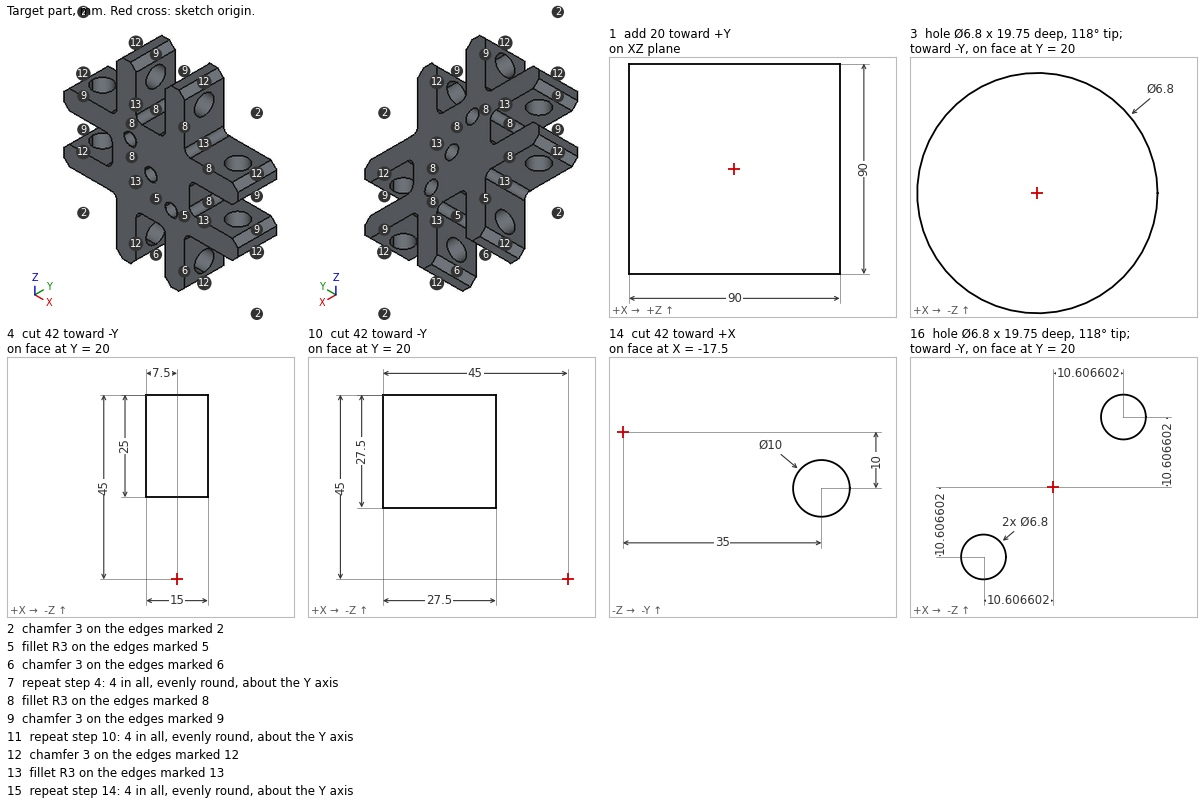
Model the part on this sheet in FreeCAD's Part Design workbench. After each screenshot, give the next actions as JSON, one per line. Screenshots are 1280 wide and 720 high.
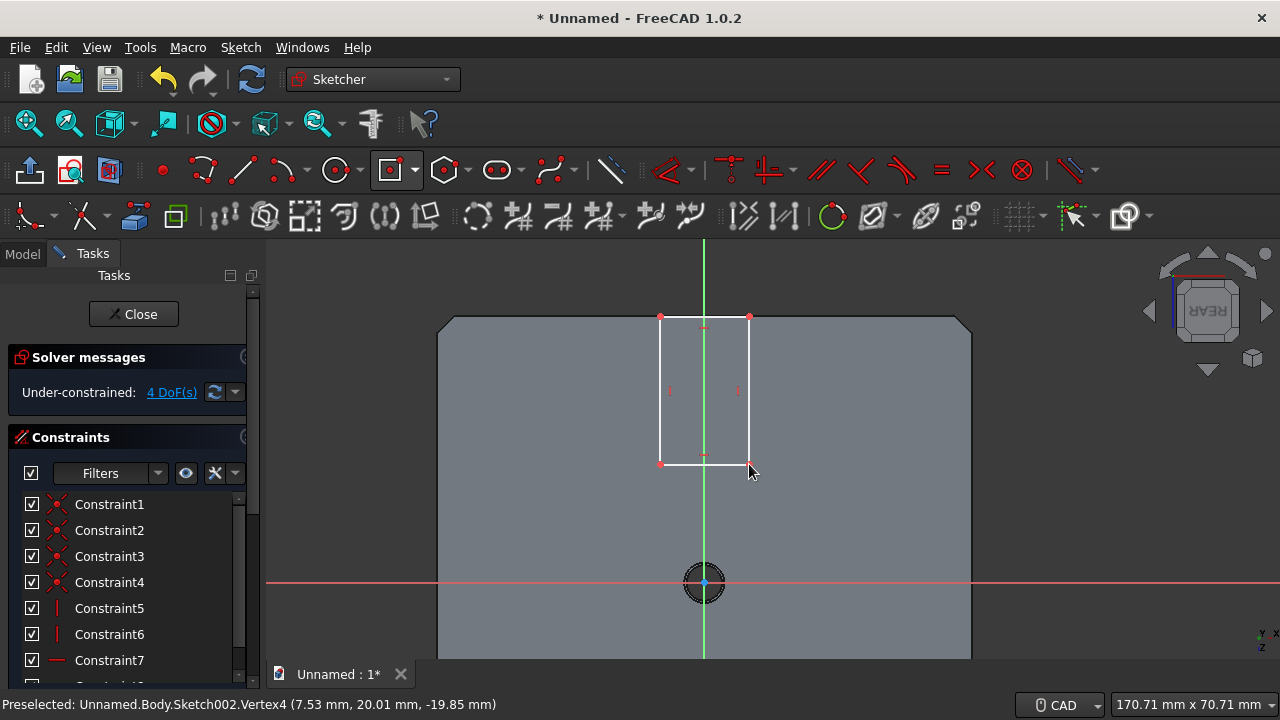
{"action": "left_click", "coordinate": [666, 170]}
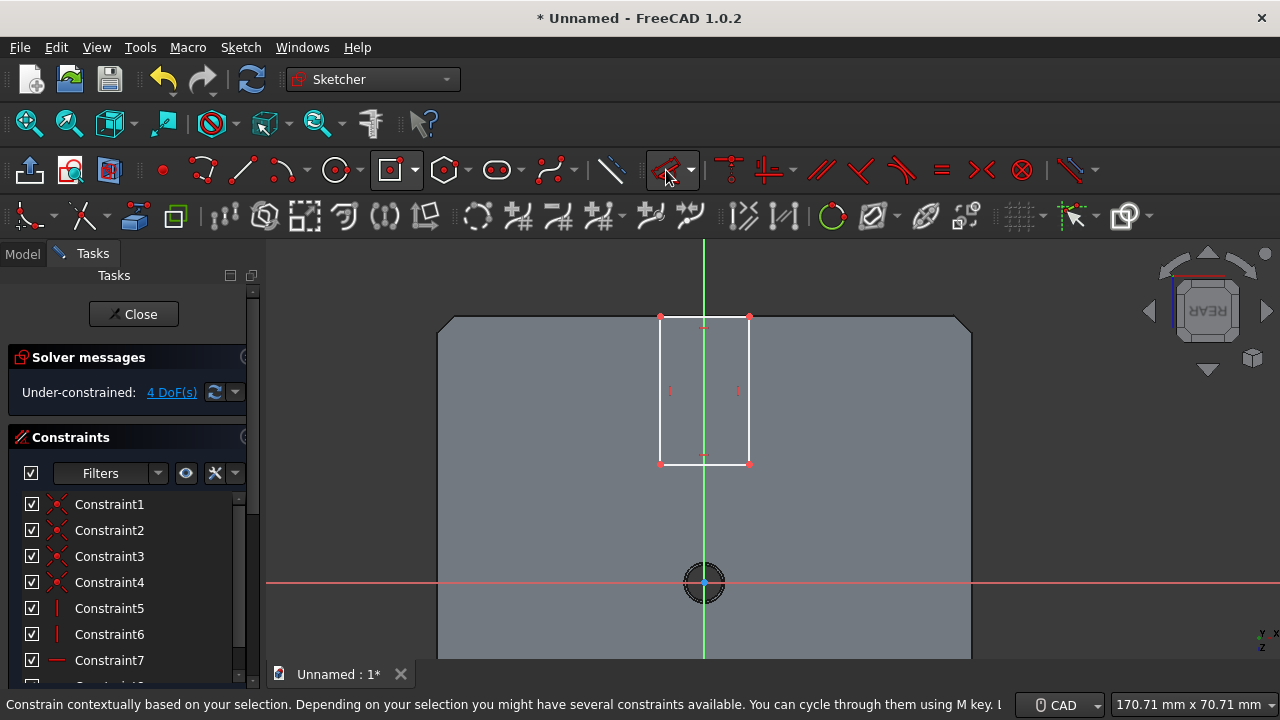
{"action": "left_click", "coordinate": [660, 361]}
{"action": "left_click", "coordinate": [626, 391]}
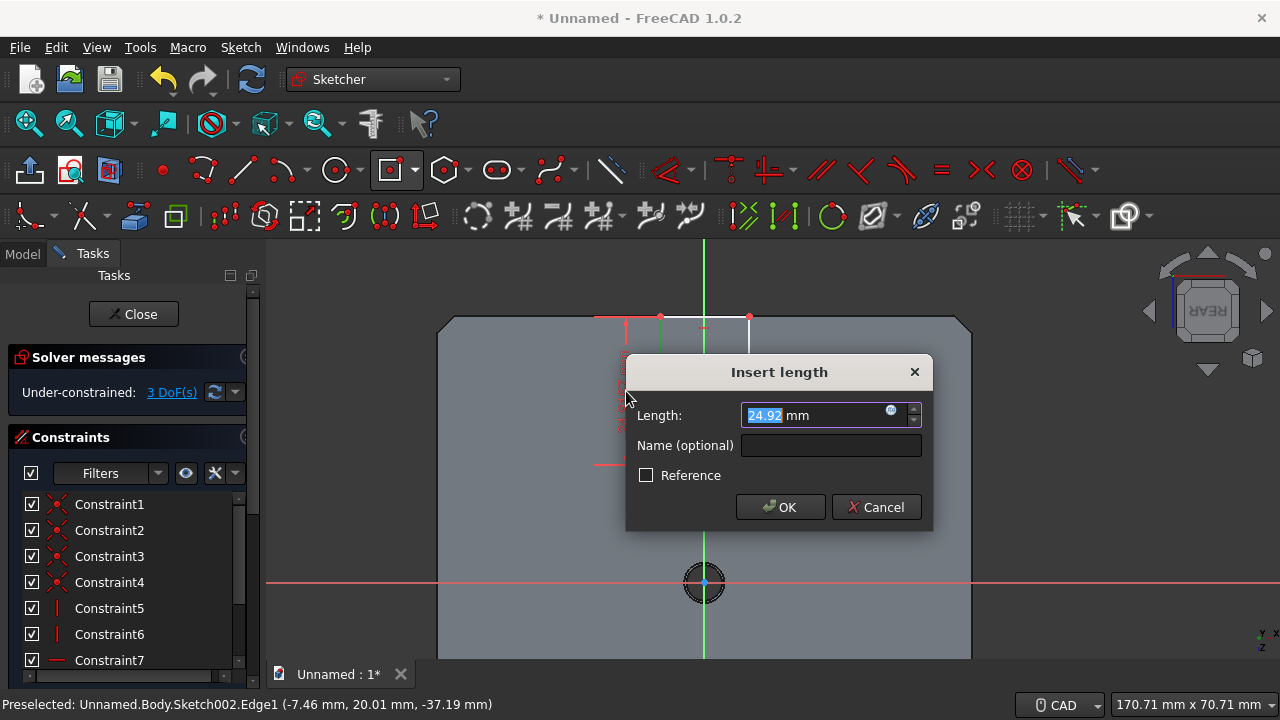
{"action": "type", "text": "25"}
{"action": "key", "text": "Return"}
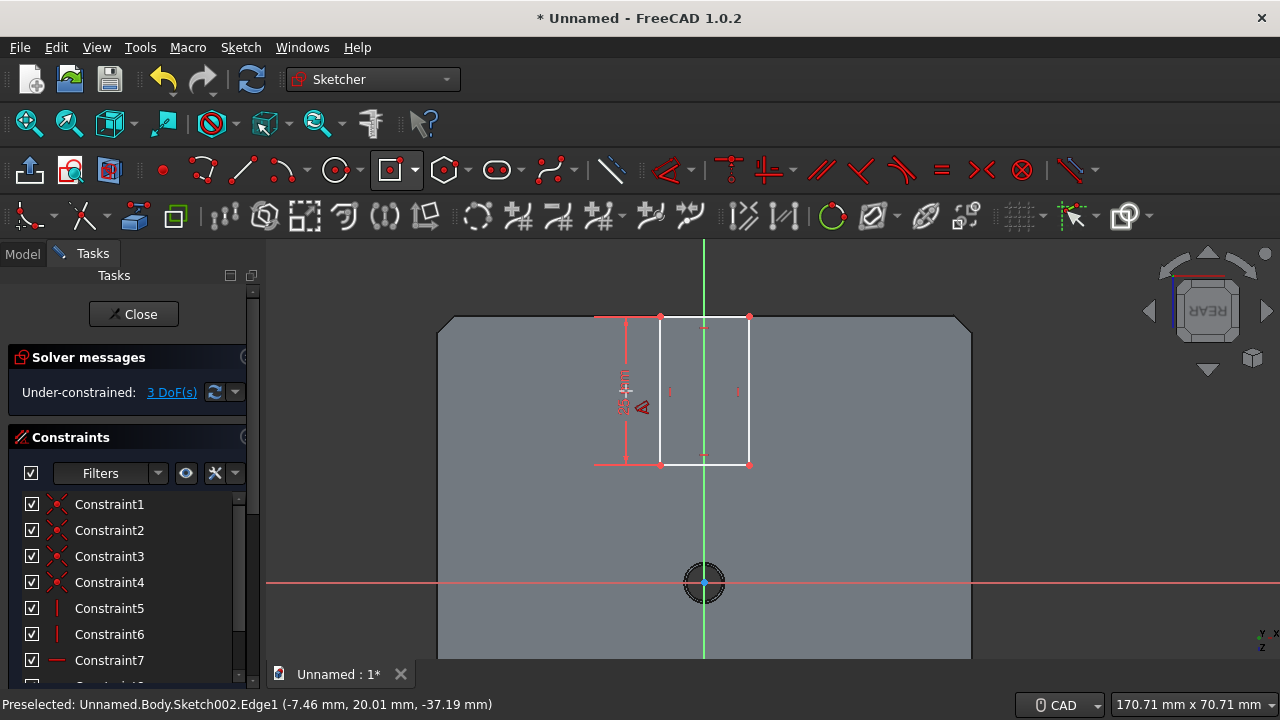
{"action": "left_click", "coordinate": [687, 465]}
{"action": "left_click", "coordinate": [684, 499]}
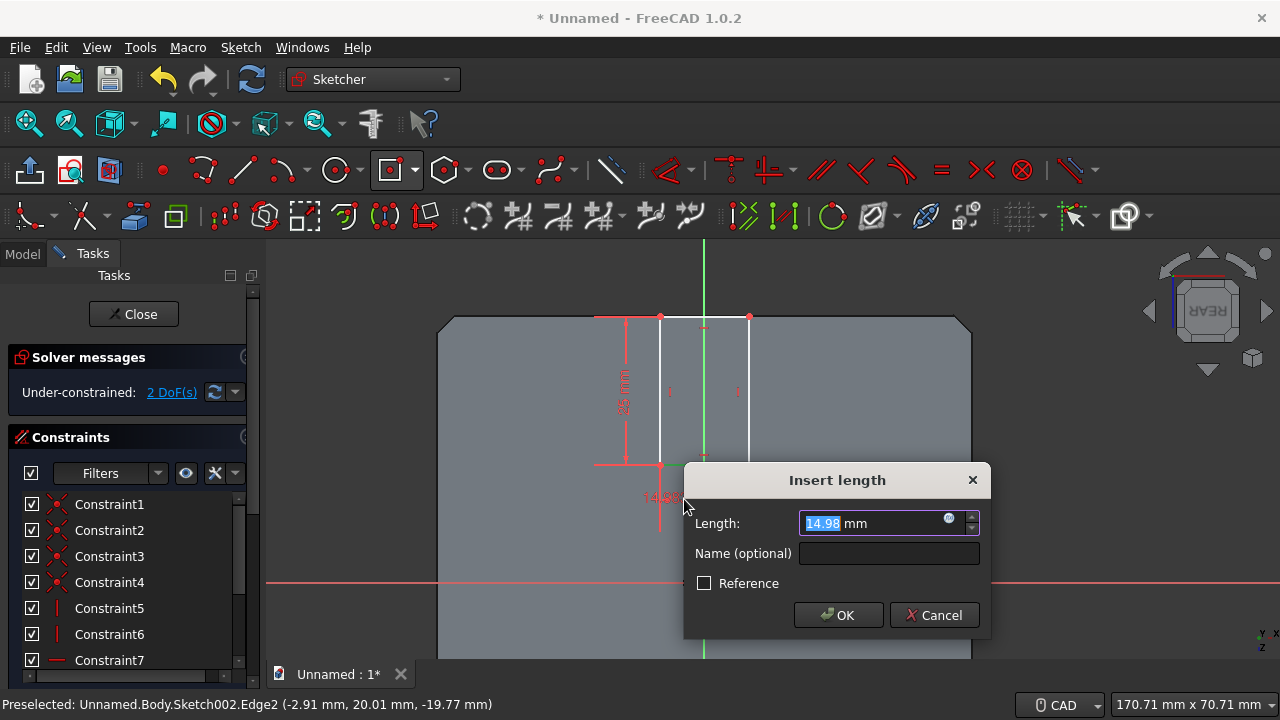
{"action": "type", "text": "15"}
{"action": "key", "text": "Return"}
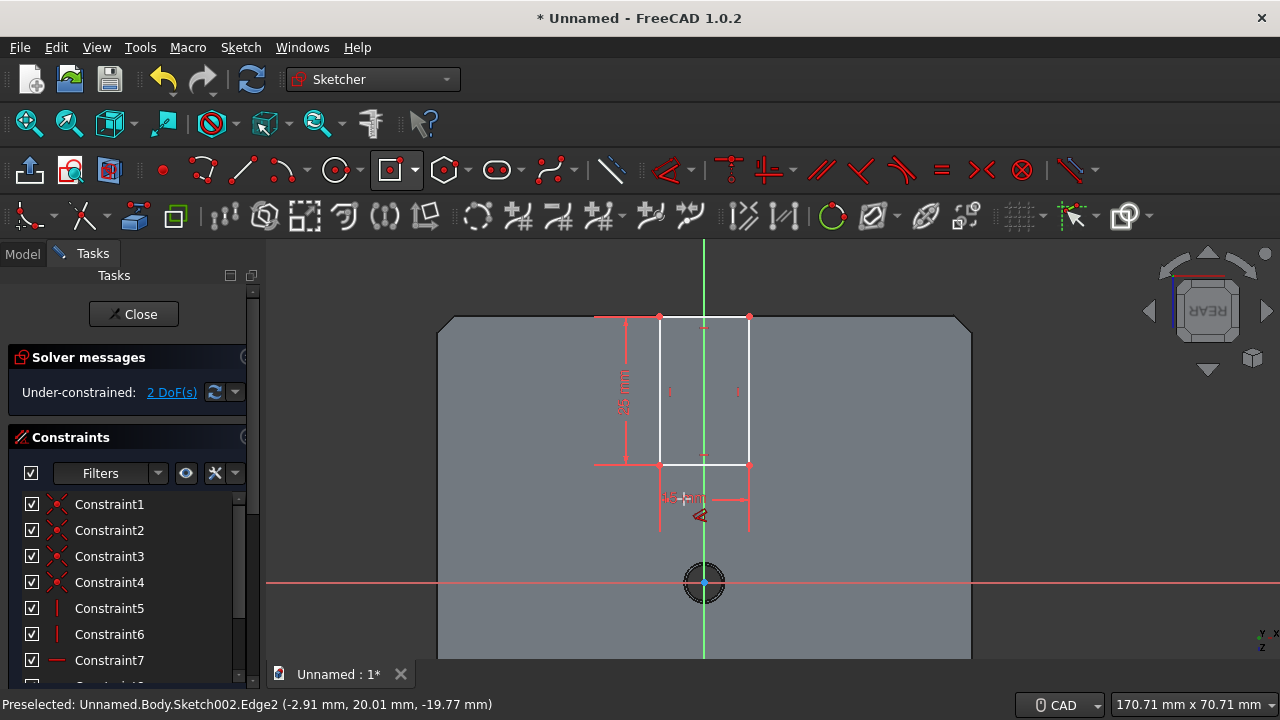
{"action": "left_click", "coordinate": [660, 317]}
{"action": "left_click", "coordinate": [626, 450]}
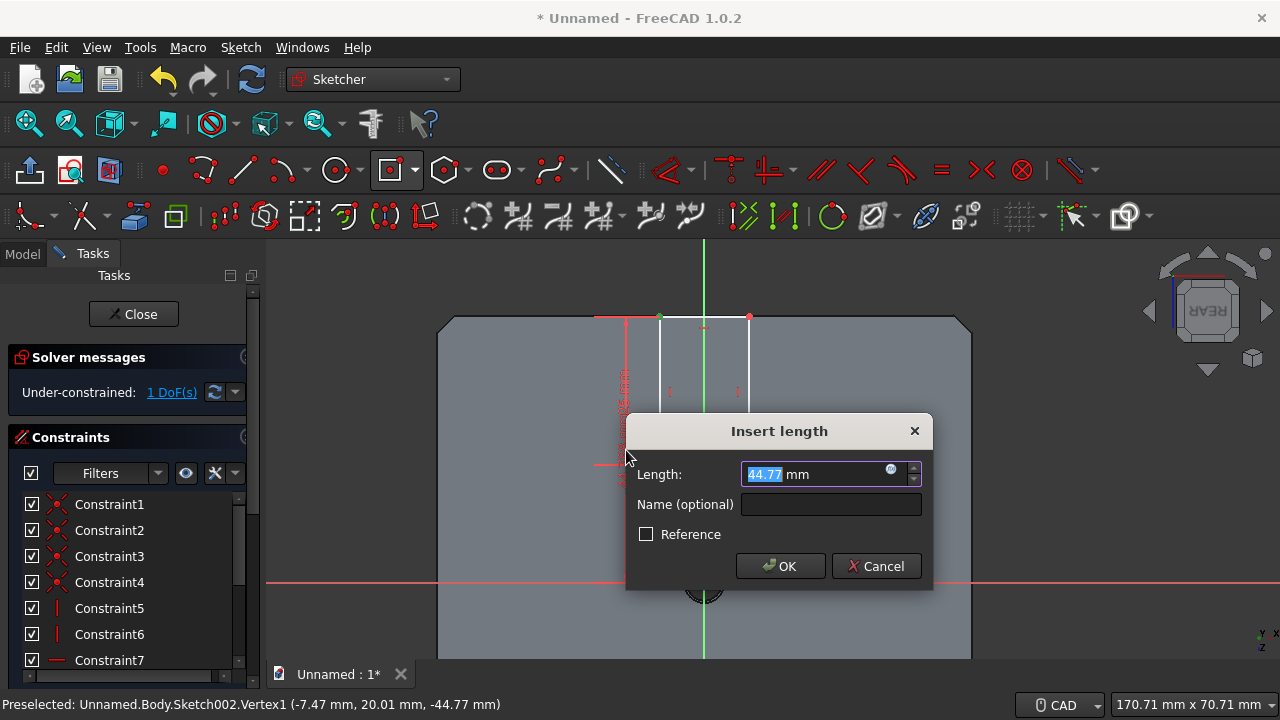
{"action": "type", "text": "45"}
{"action": "key", "text": "Return"}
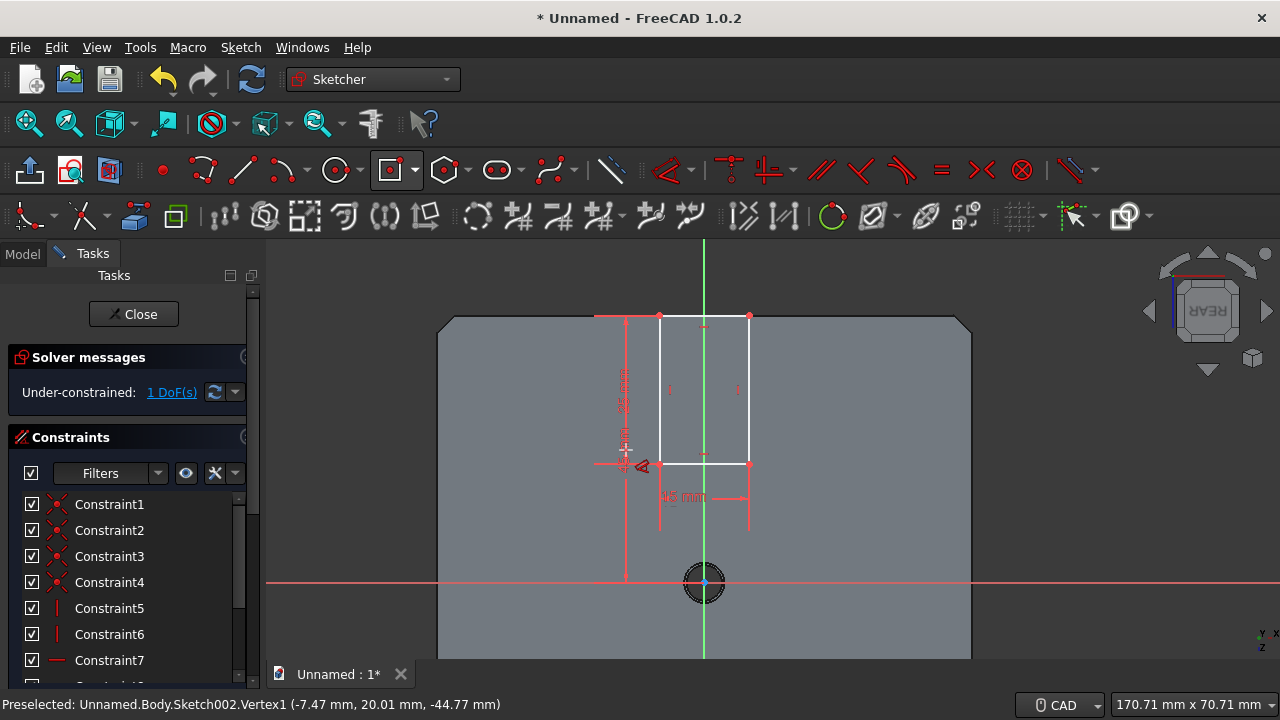
{"action": "left_click", "coordinate": [660, 316]}
{"action": "left_click", "coordinate": [682, 617]}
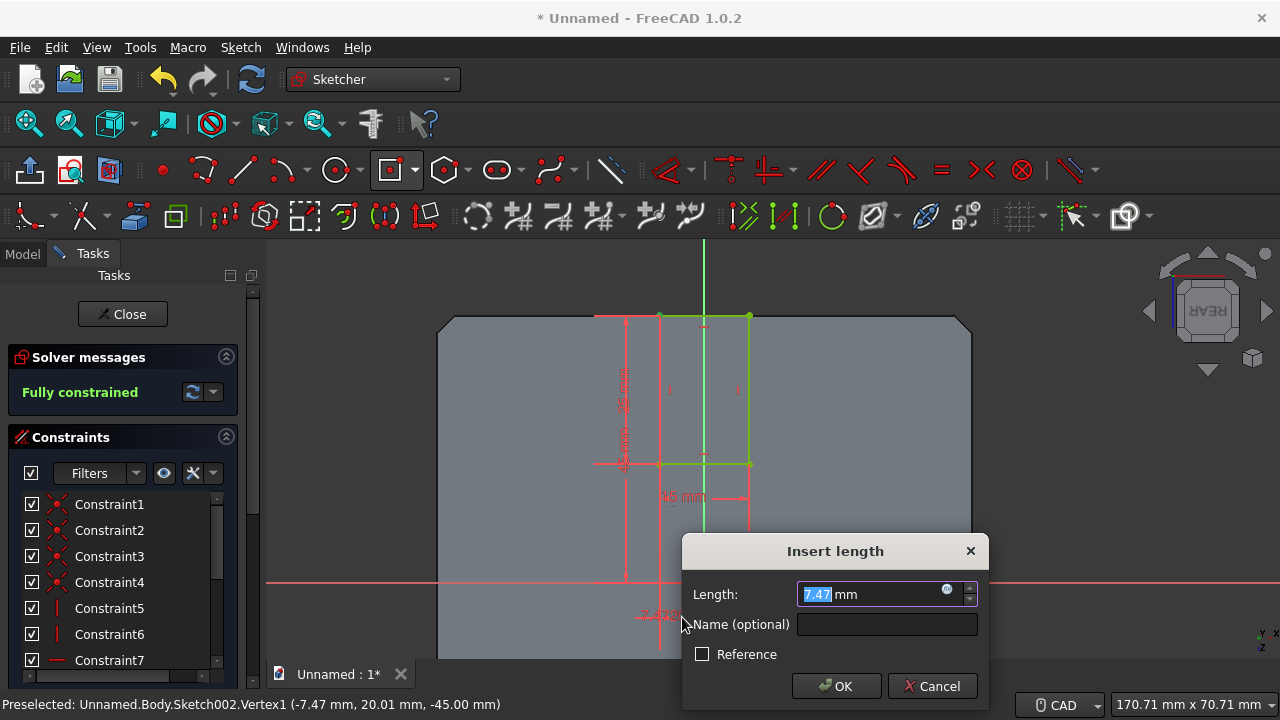
{"action": "type", "text": "7.5"}
{"action": "key", "text": "Return"}
{"action": "key", "text": "Escape"}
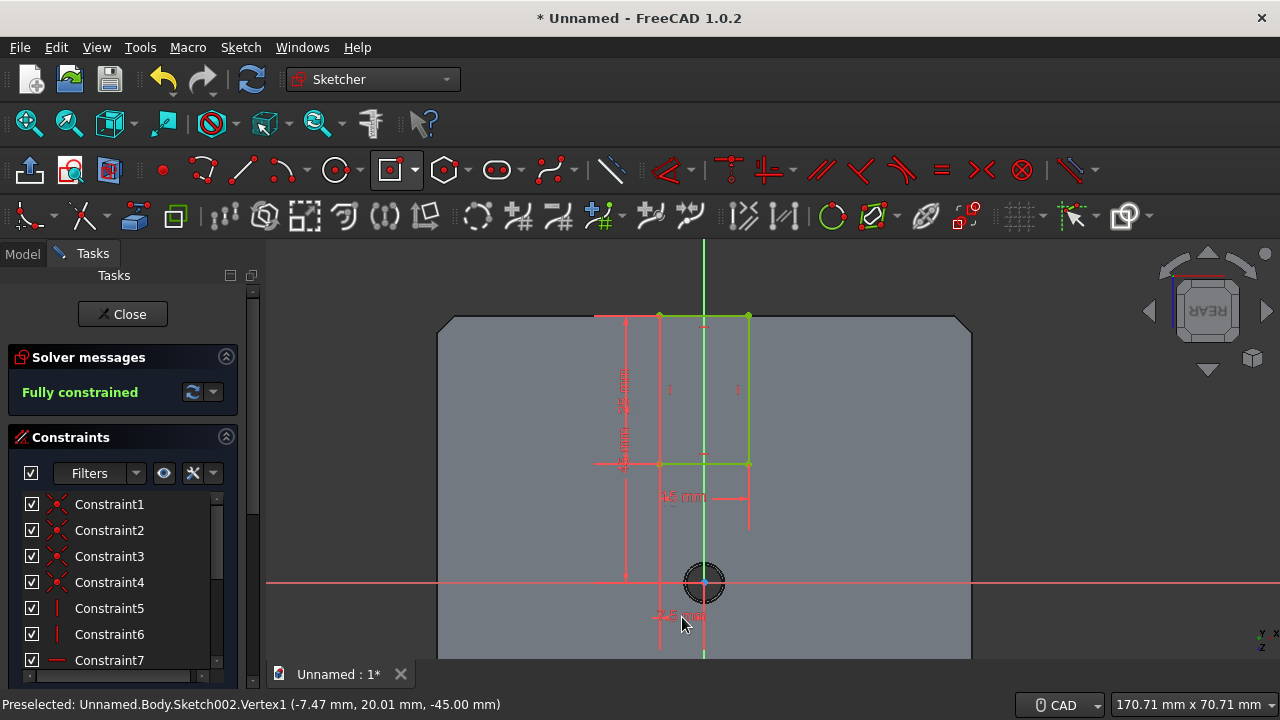
{"action": "left_click", "coordinate": [123, 314]}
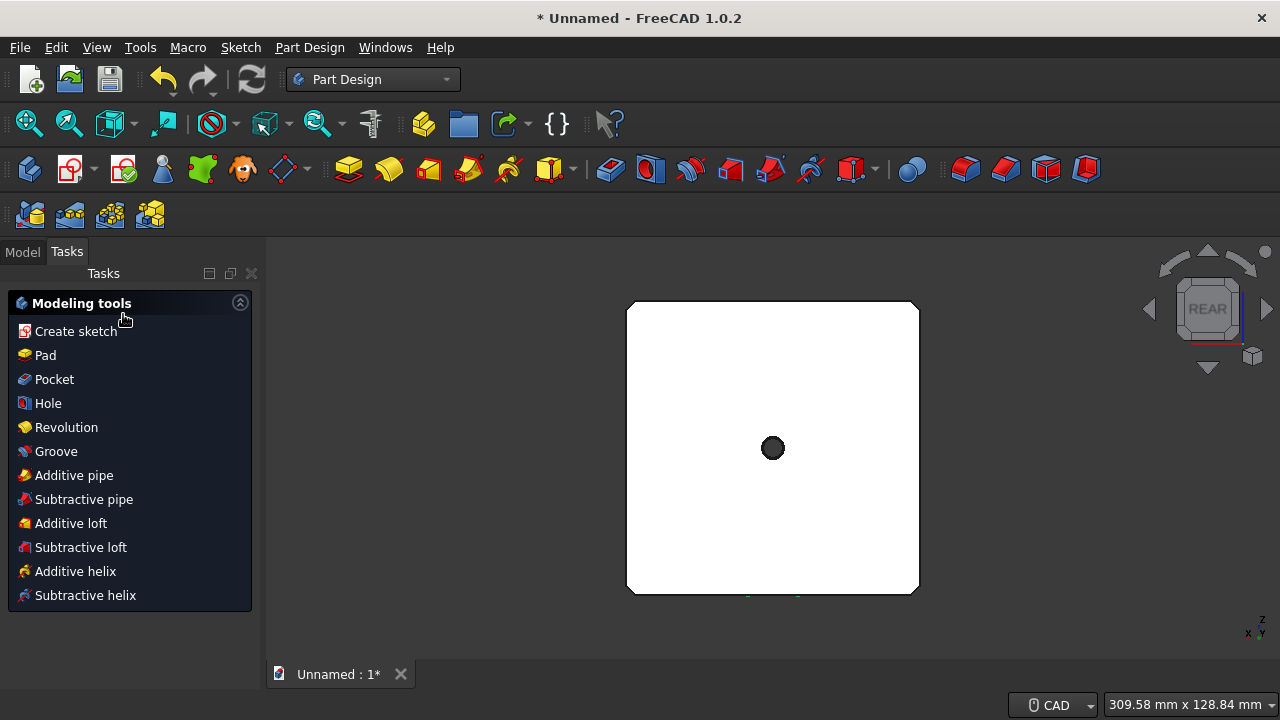
{"action": "left_click", "coordinate": [612, 170]}